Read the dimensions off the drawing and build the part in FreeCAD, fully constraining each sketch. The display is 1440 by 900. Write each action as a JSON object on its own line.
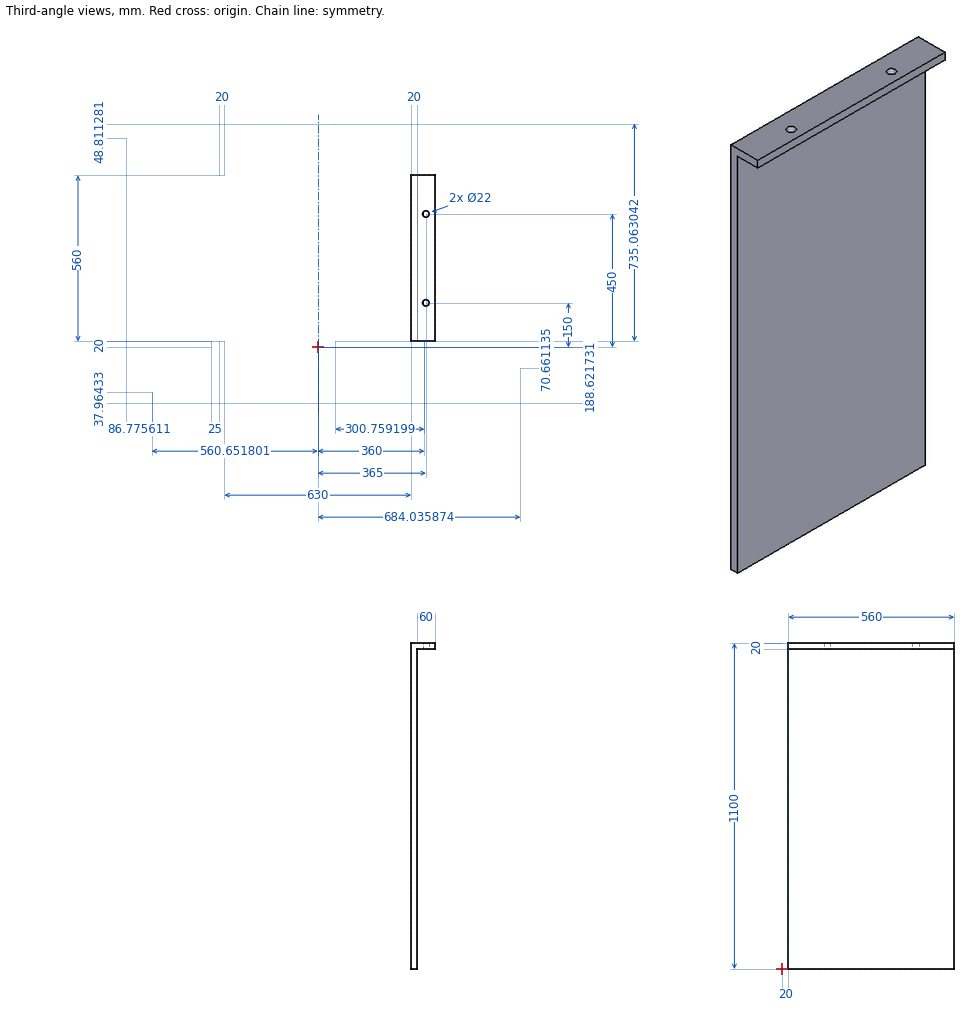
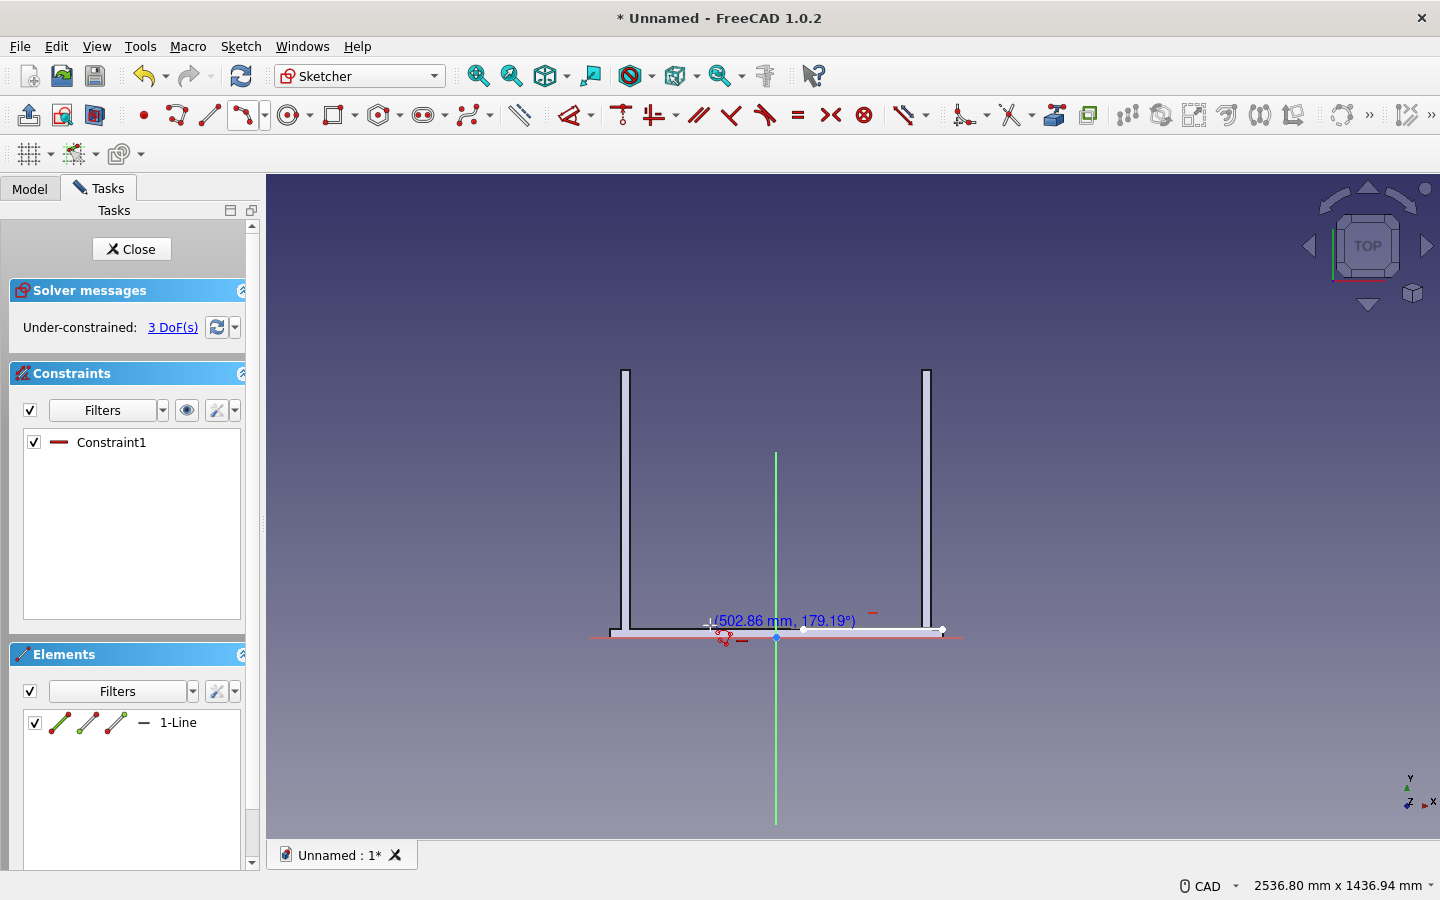
{"action": "left_click", "coordinate": [1093, 671]}
{"action": "left_click", "coordinate": [943, 725]}
{"action": "left_click", "coordinate": [517, 704]}
{"action": "left_click", "coordinate": [477, 311]}
{"action": "left_click", "coordinate": [804, 289]}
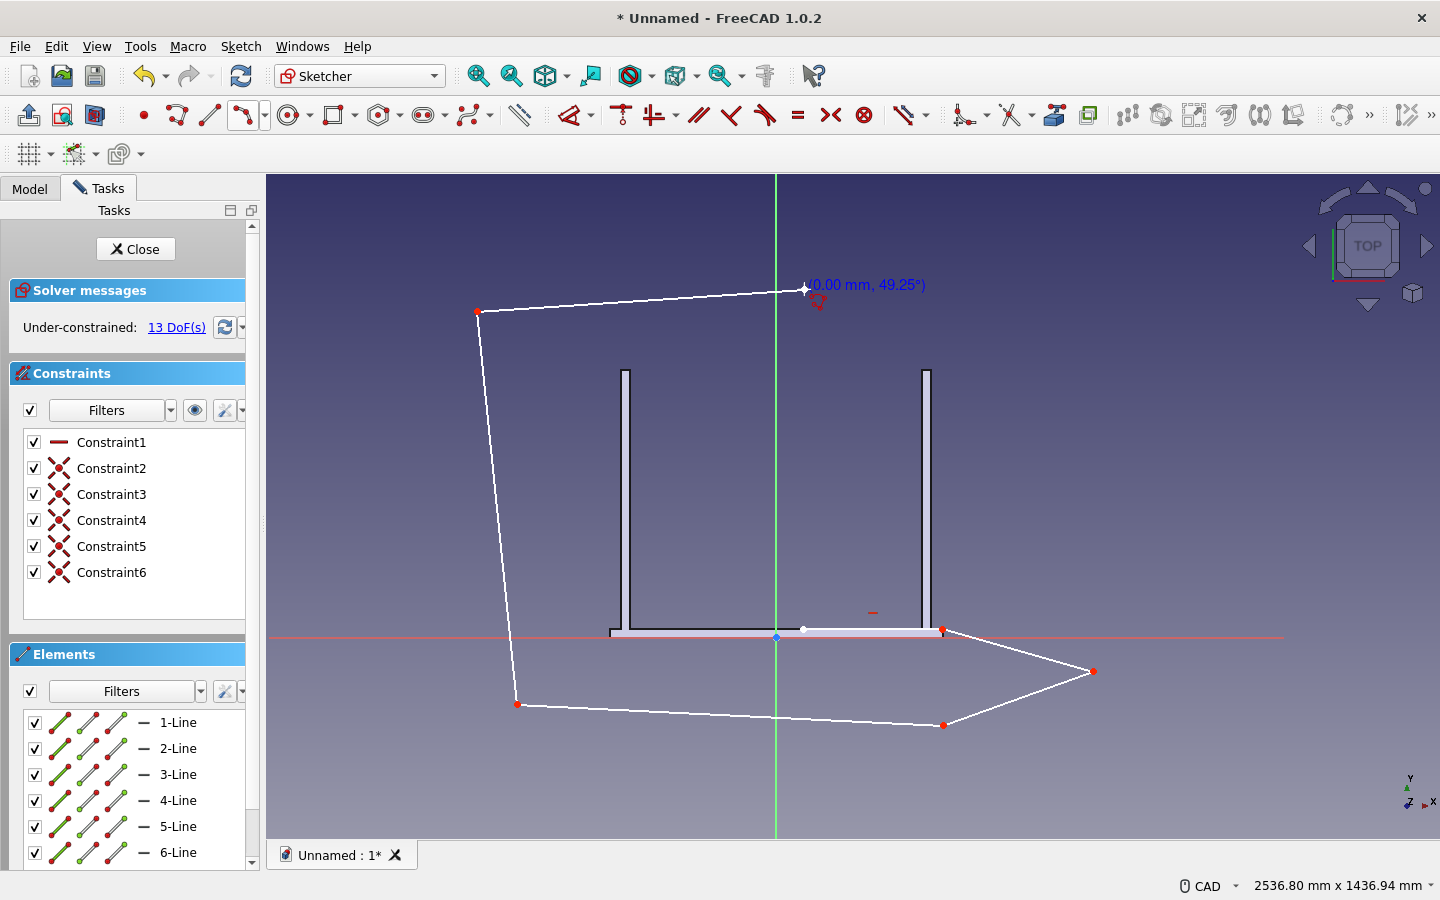
{"action": "scroll", "coordinate": [804, 629], "scroll_direction": "up", "scroll_amount": 3}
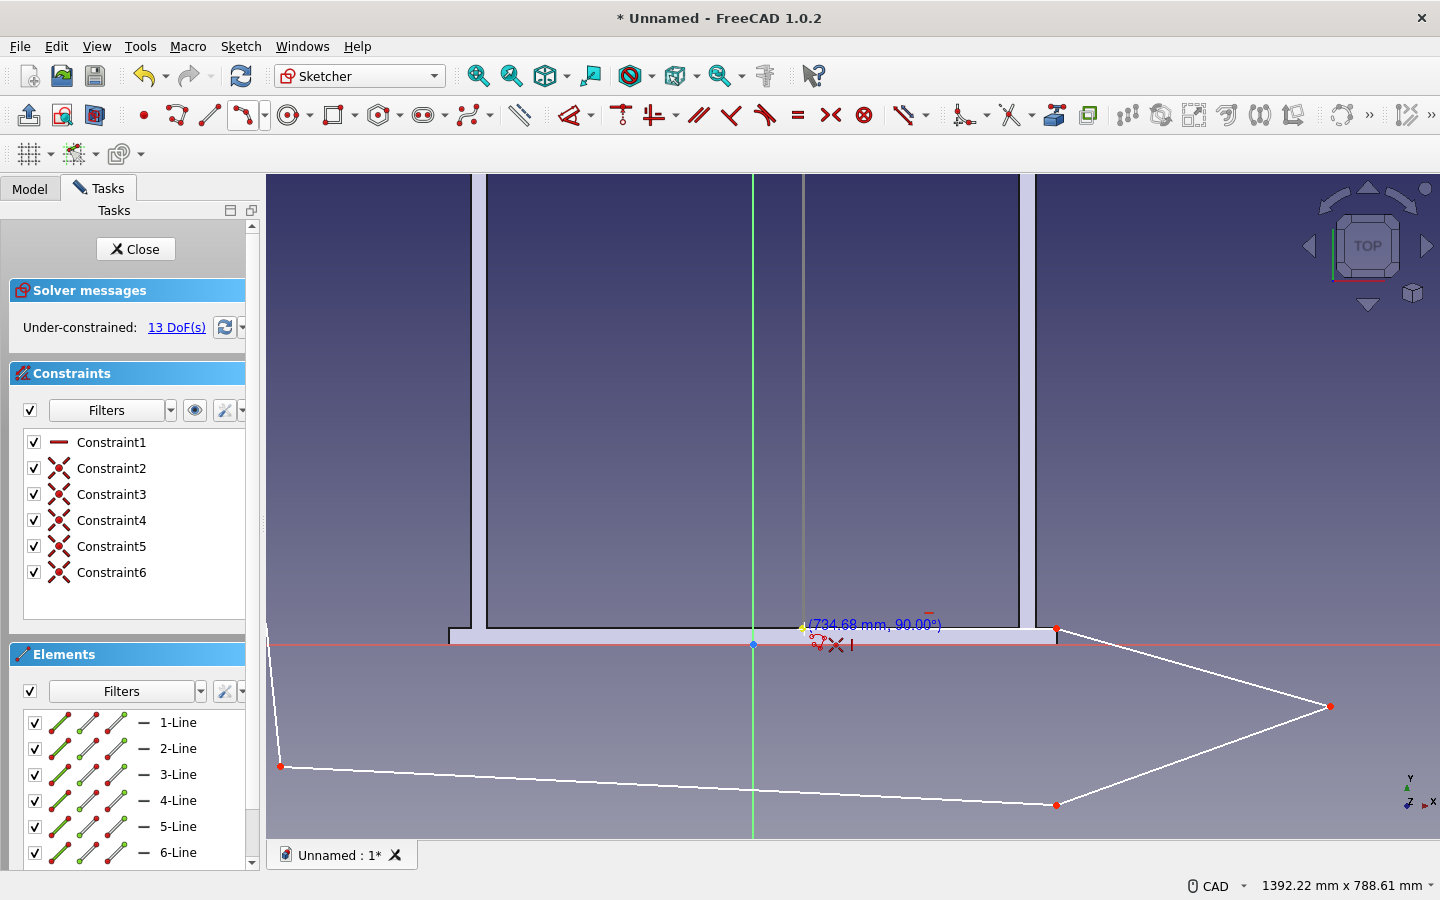
{"action": "left_click", "coordinate": [803, 629]}
{"action": "key", "text": "Escape"}
{"action": "key", "text": "Escape"}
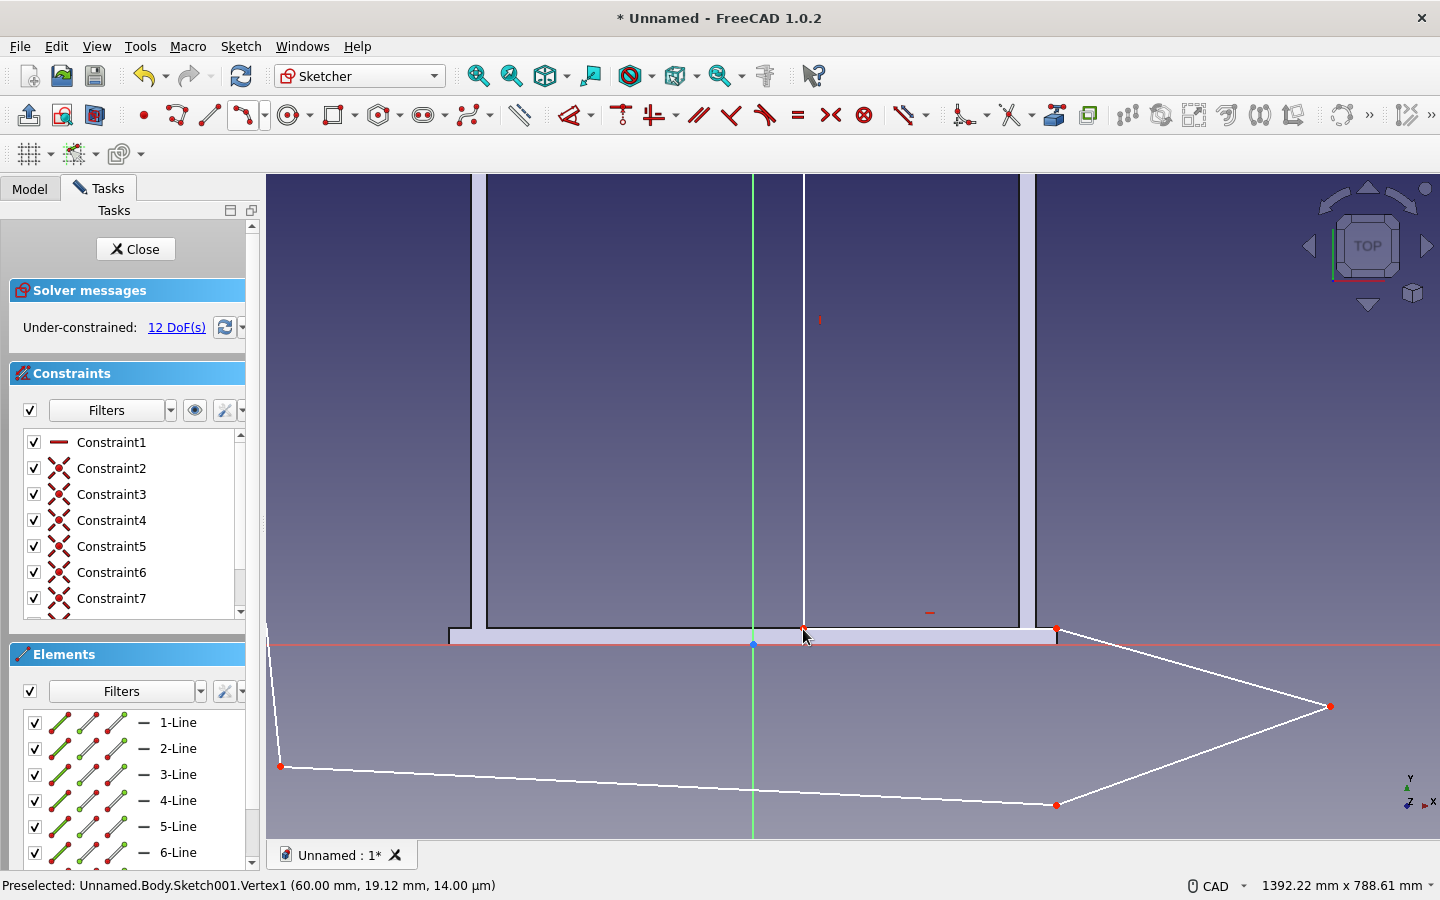
{"action": "key", "text": "d"}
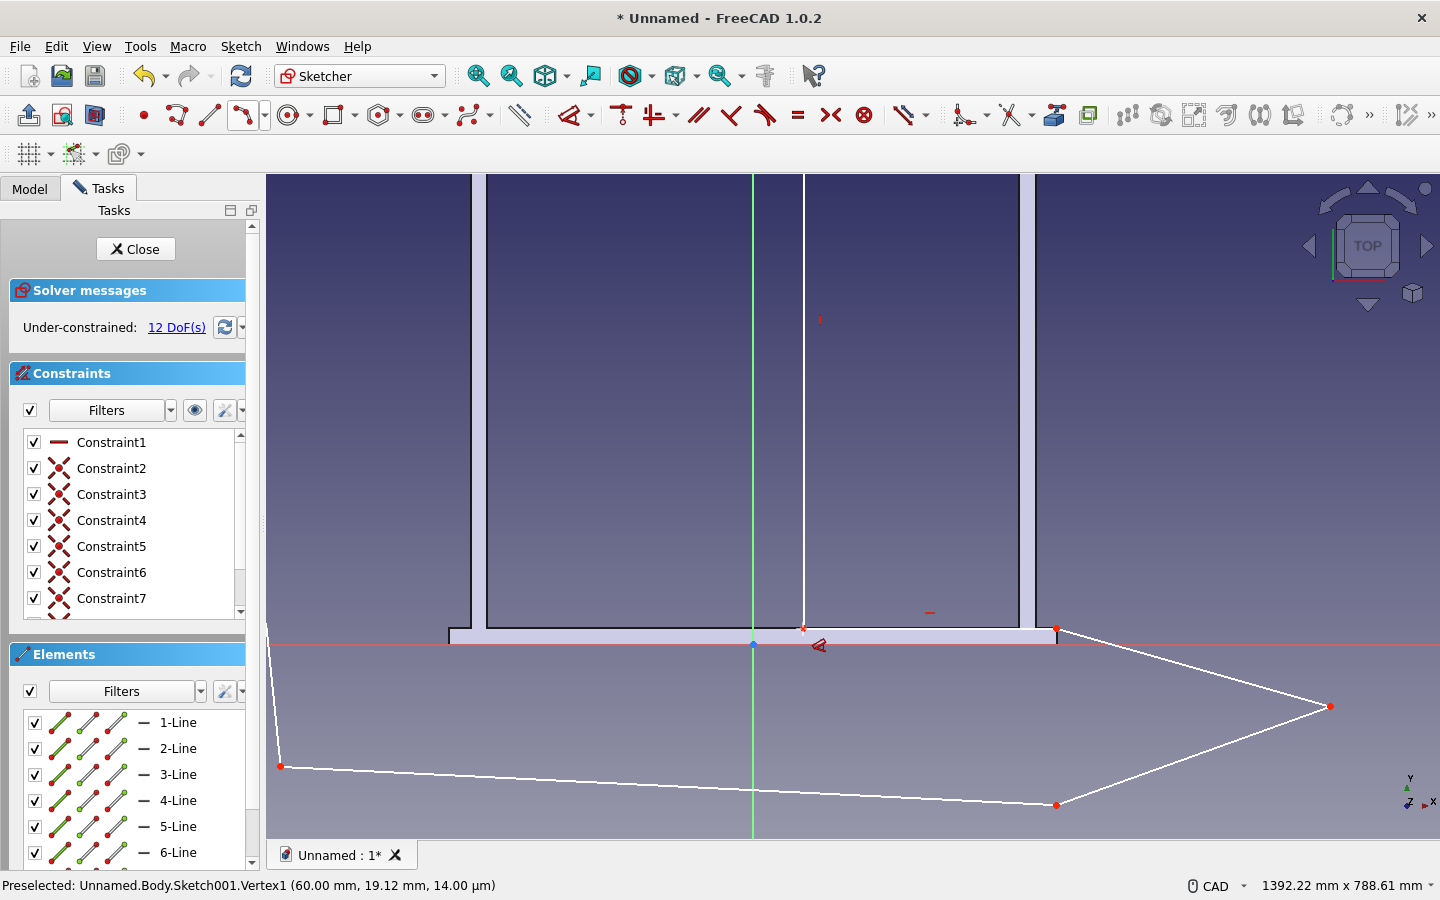
{"action": "scroll", "coordinate": [804, 629], "scroll_direction": "up", "scroll_amount": 5}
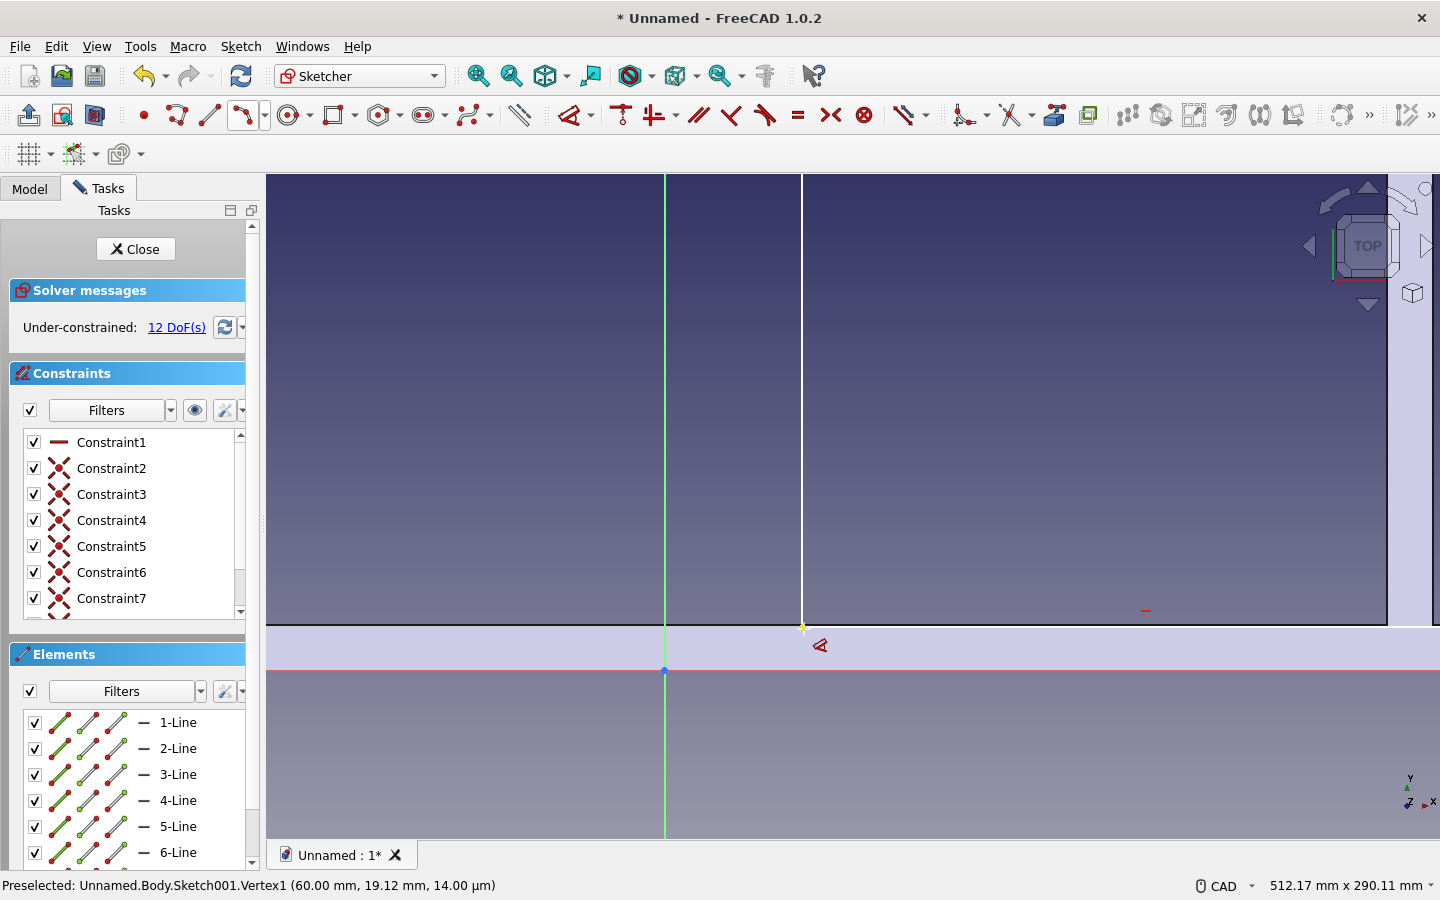
{"action": "left_click", "coordinate": [802, 627]}
{"action": "left_click", "coordinate": [836, 649]}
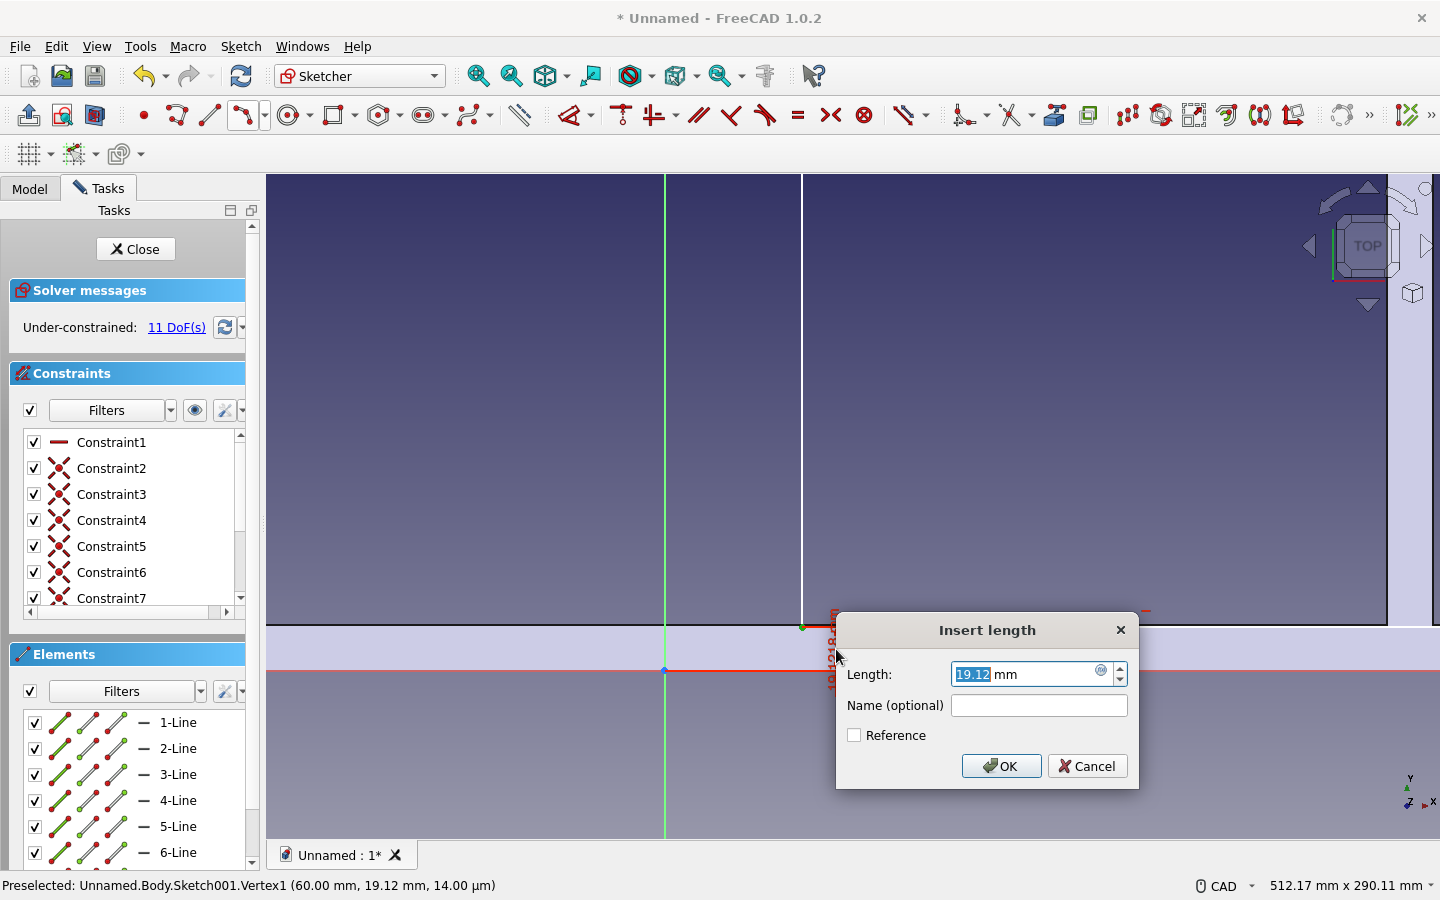
{"action": "type", "text": "20"}
{"action": "key", "text": "Return"}